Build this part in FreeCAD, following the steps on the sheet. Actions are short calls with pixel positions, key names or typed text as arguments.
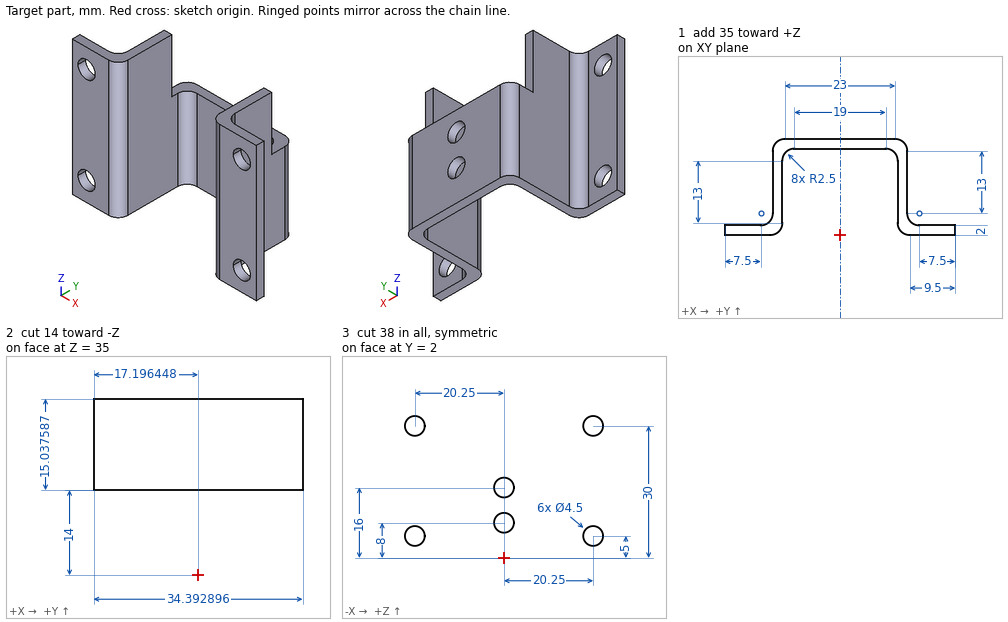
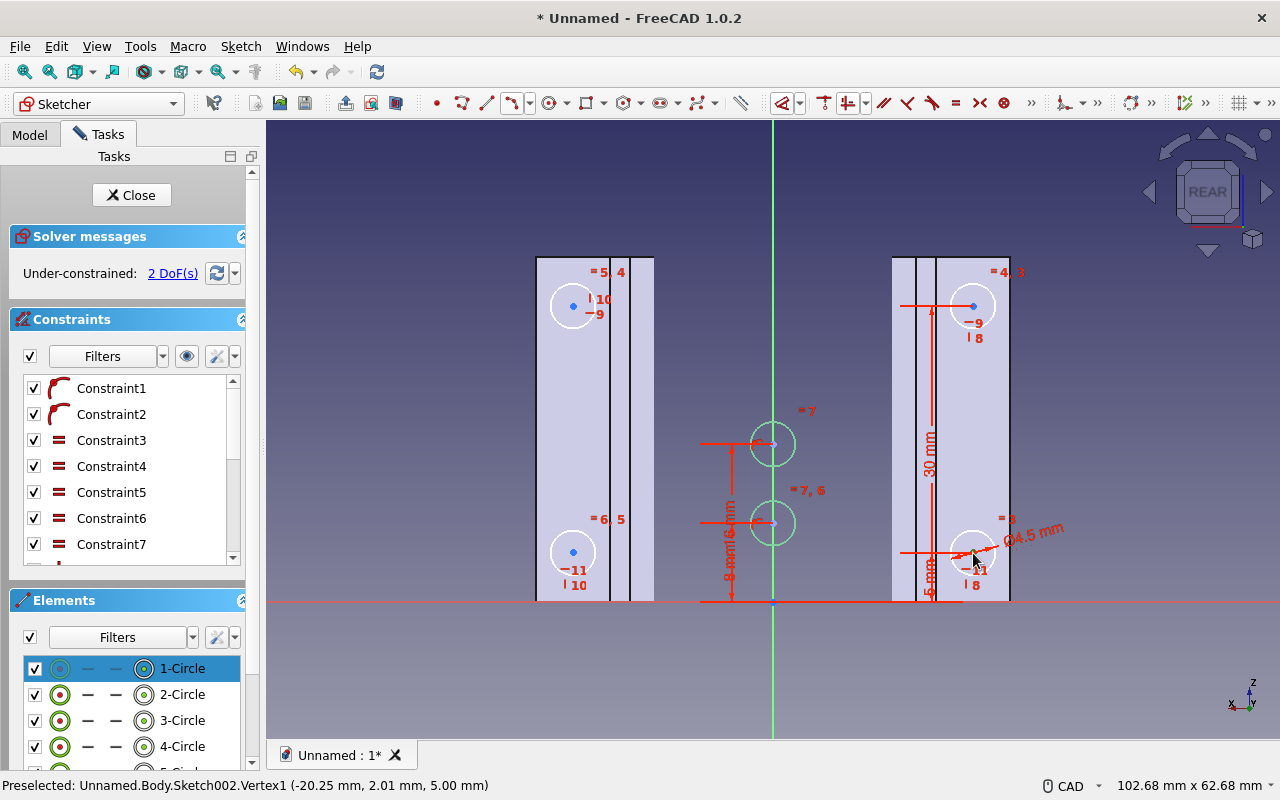
key(l)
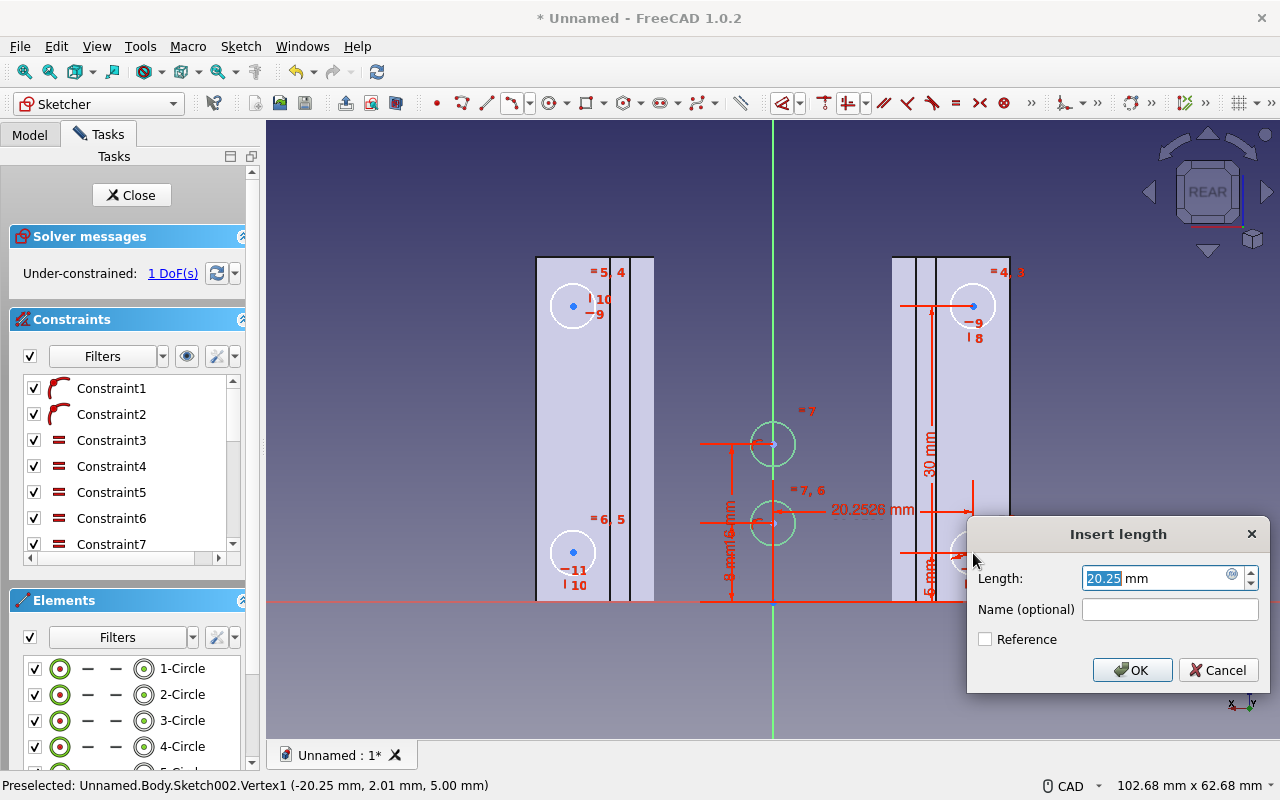
text(20.25)
key(Return)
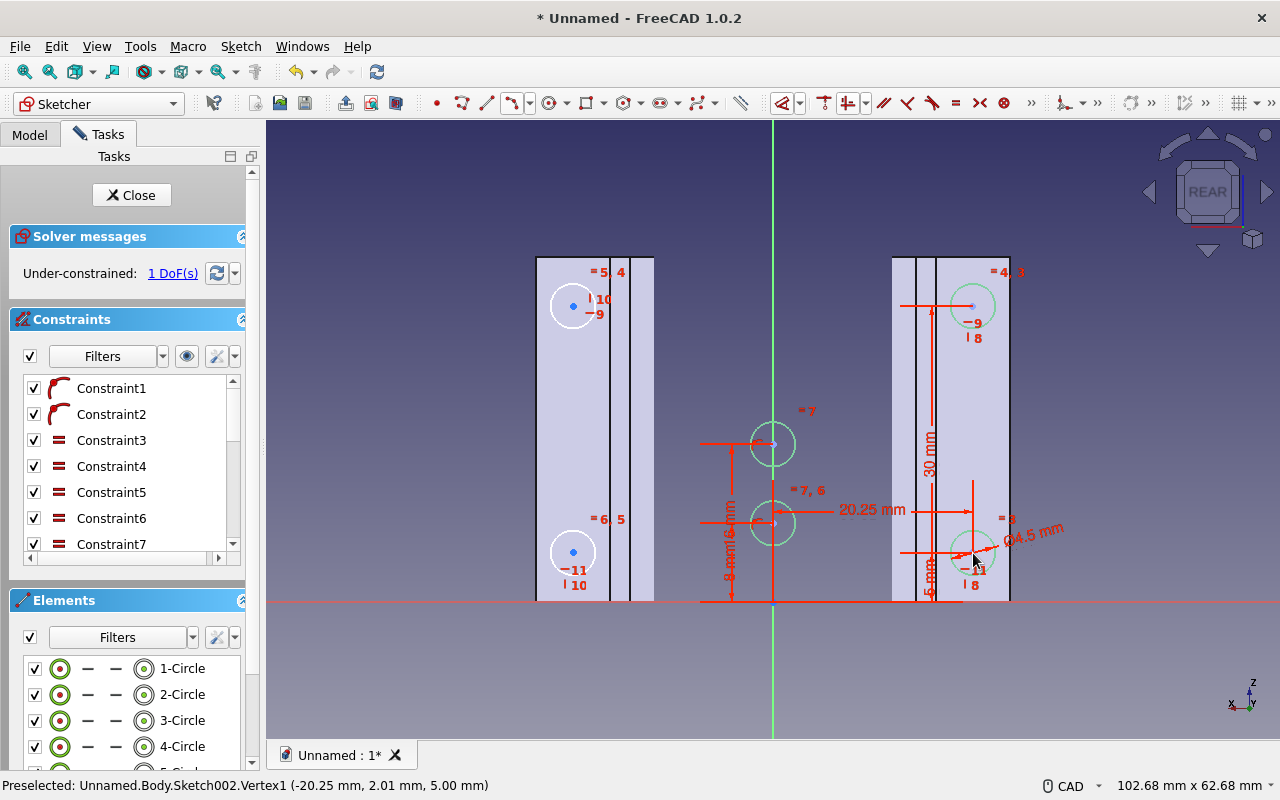
click(573, 306)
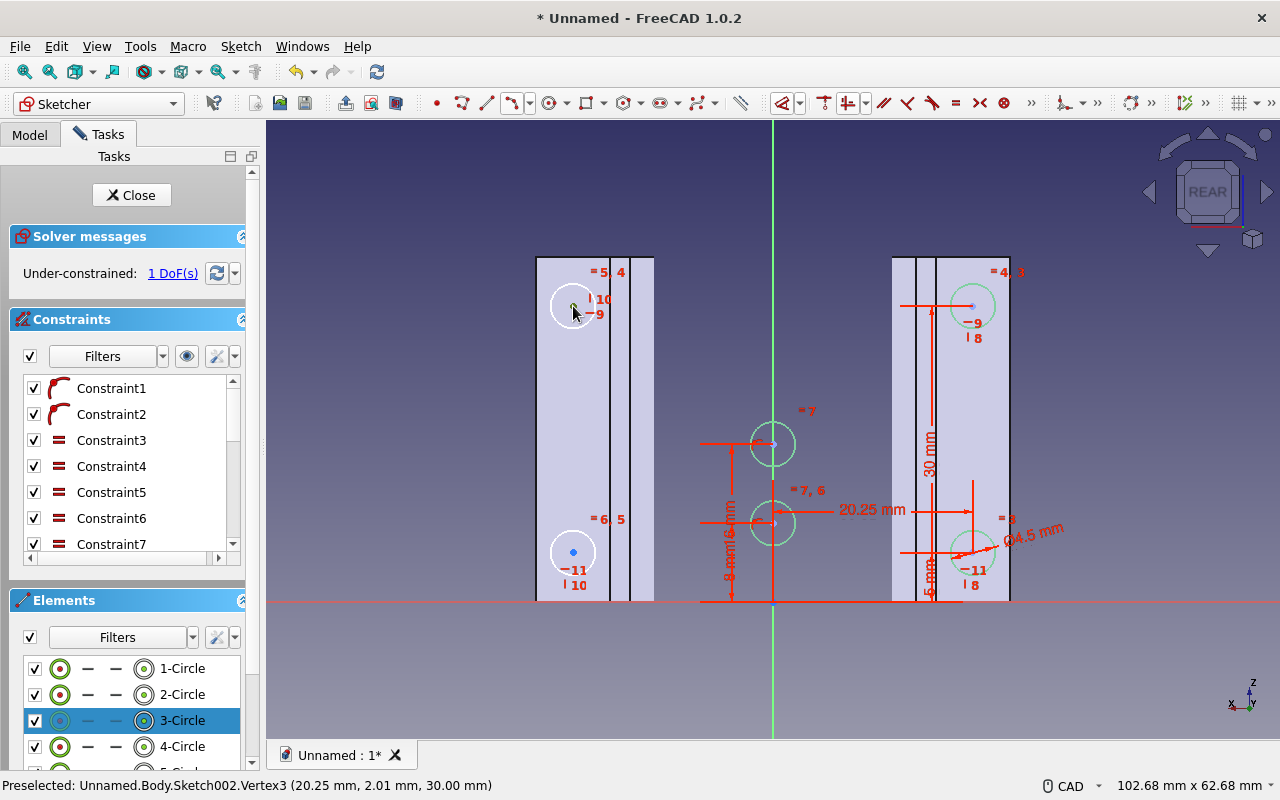
key(l)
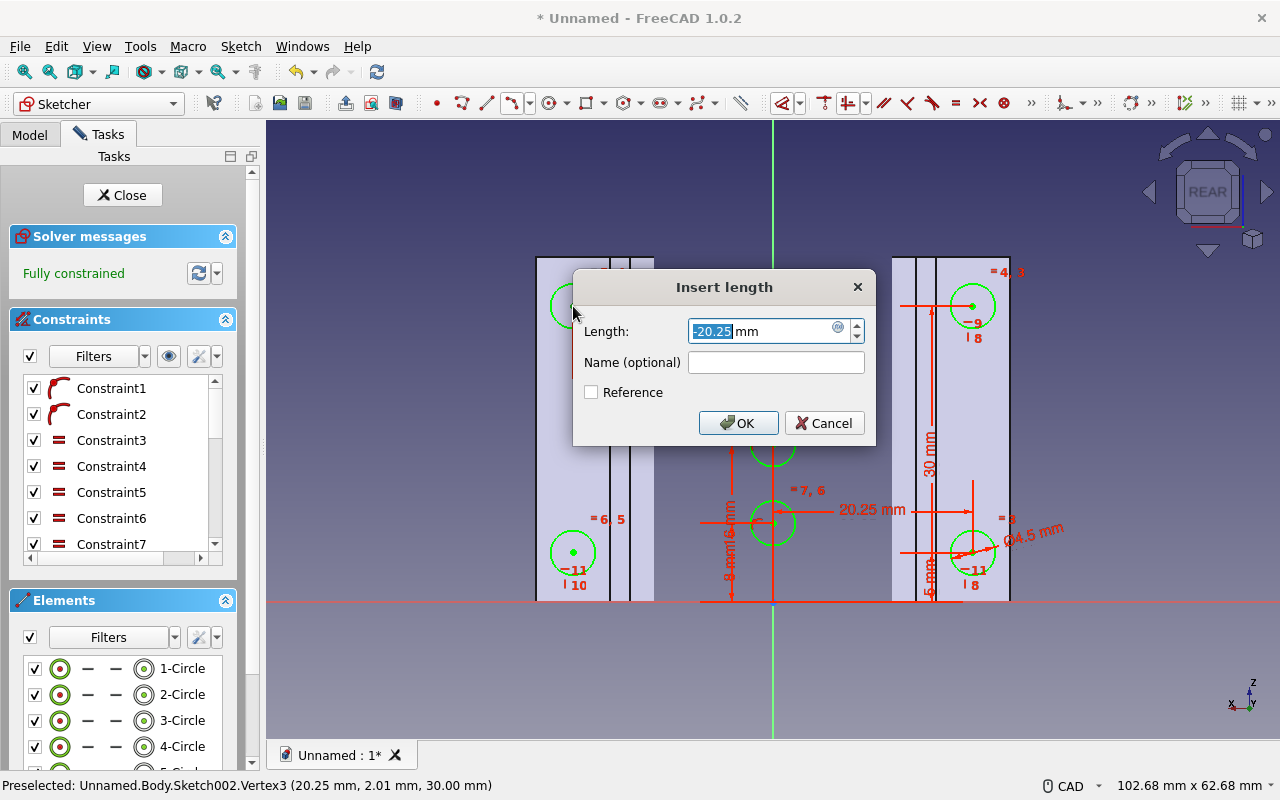
text(-20.25)
key(Return)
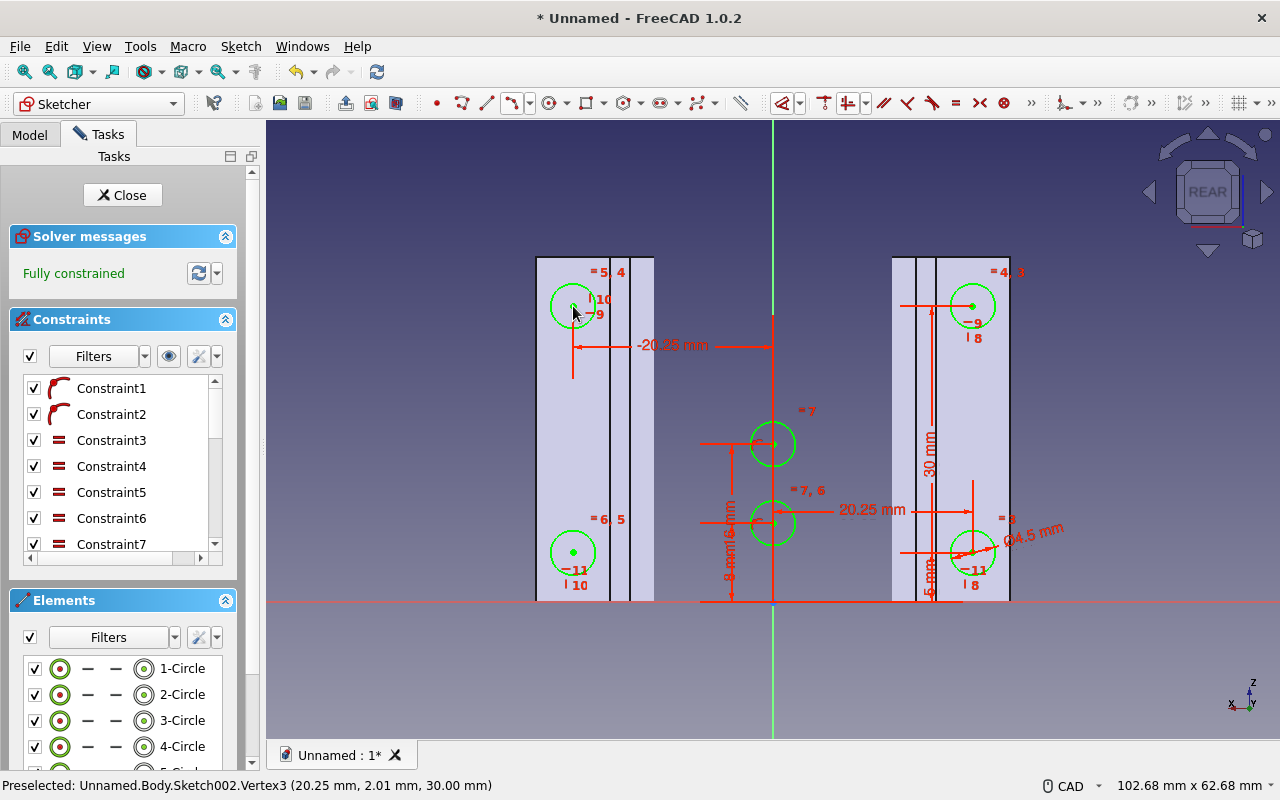
click(123, 195)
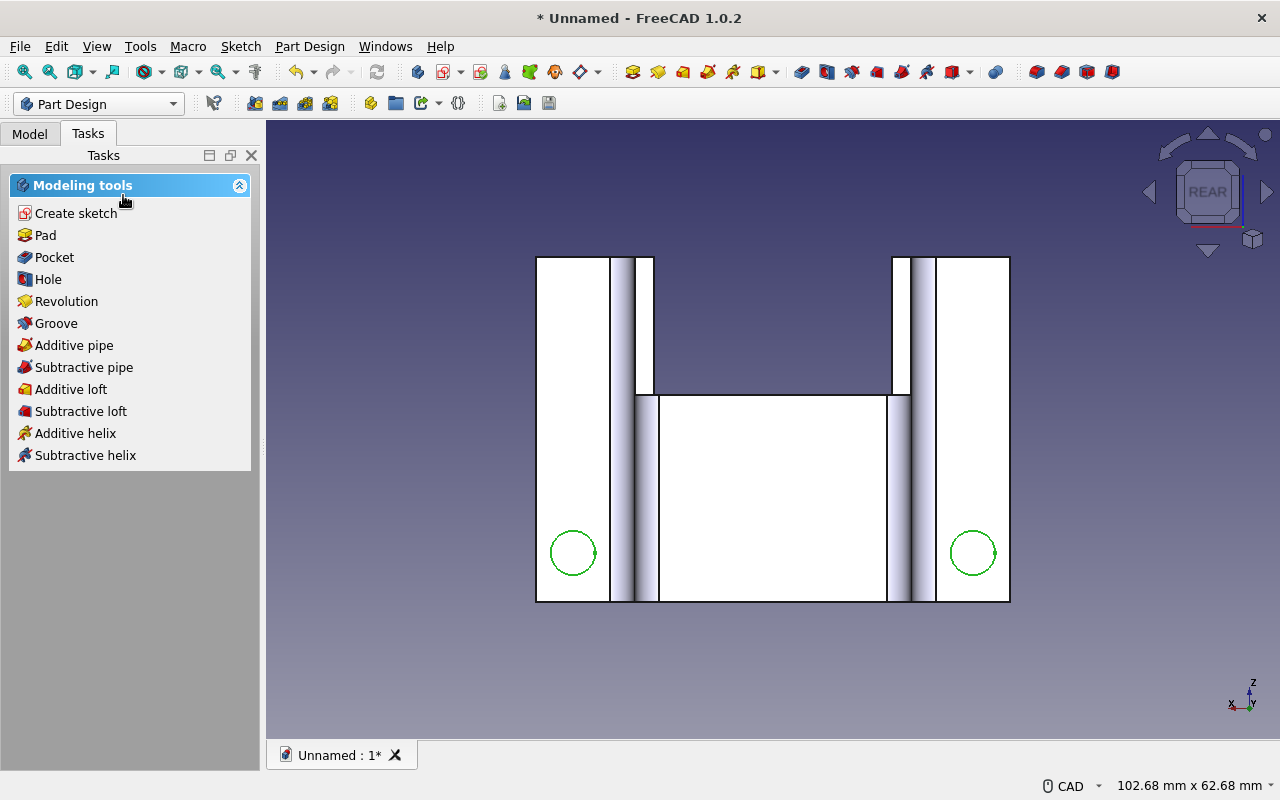
click(802, 72)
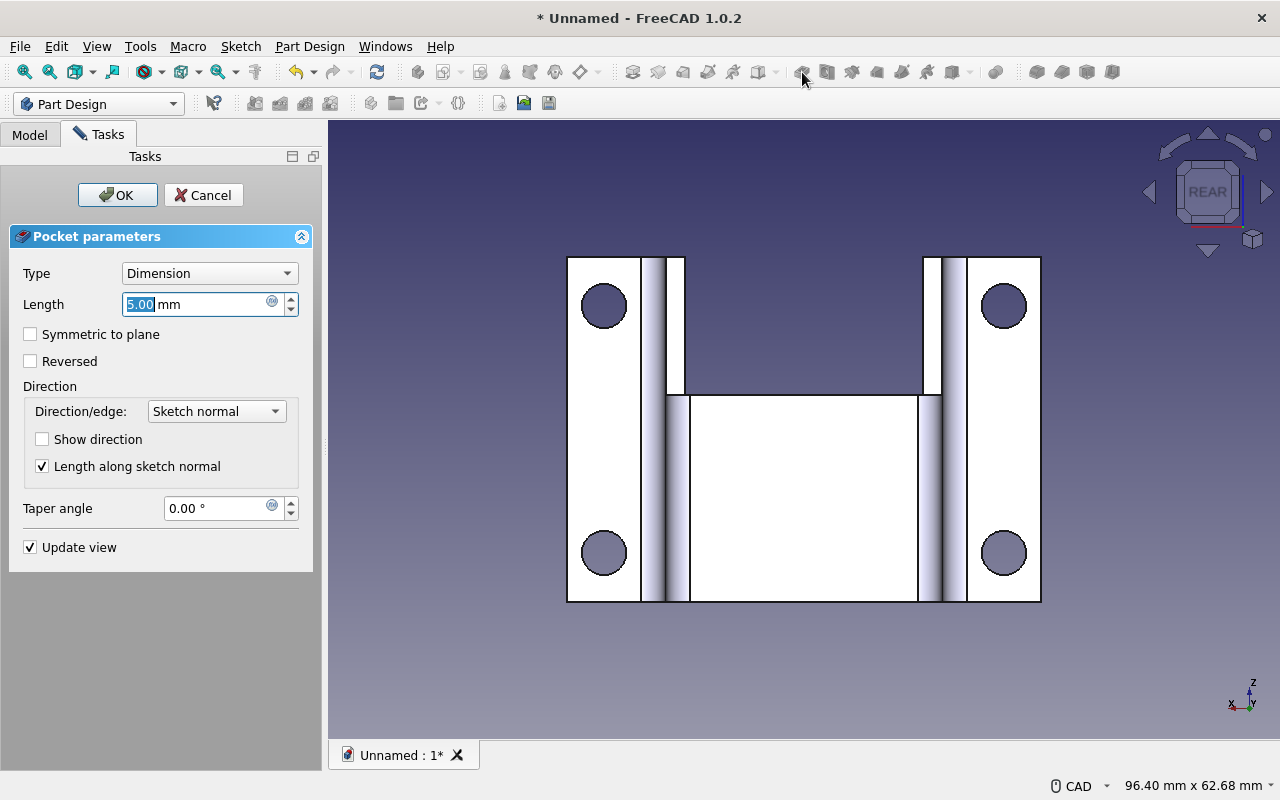
text(38)
key(Tab)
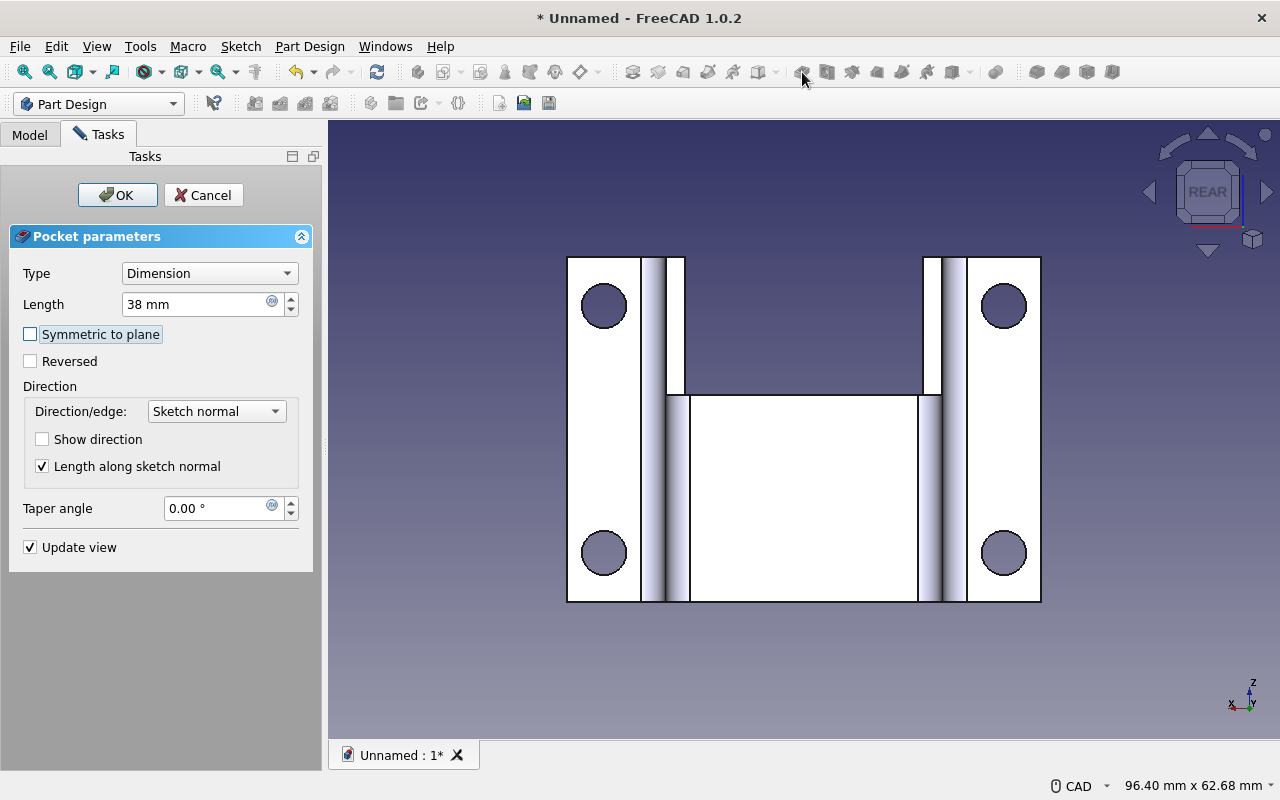
click(31, 334)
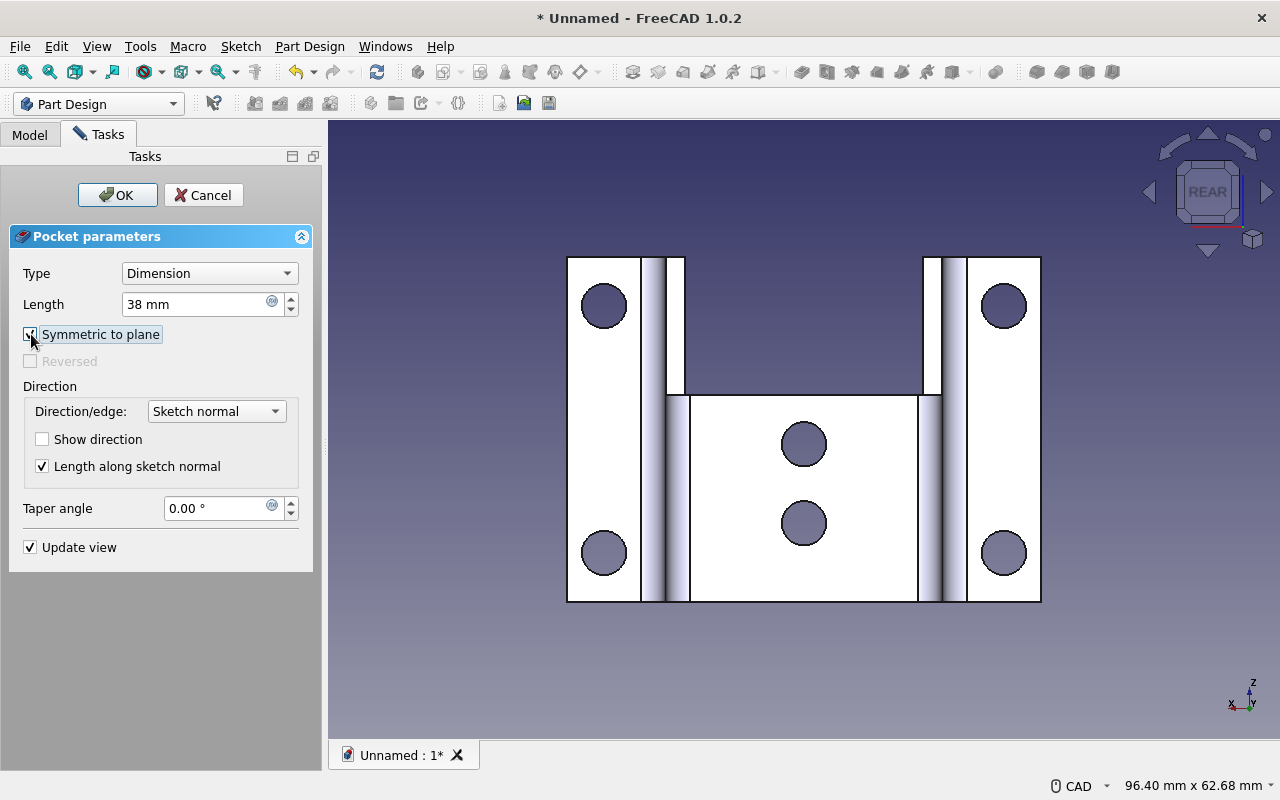
click(118, 195)